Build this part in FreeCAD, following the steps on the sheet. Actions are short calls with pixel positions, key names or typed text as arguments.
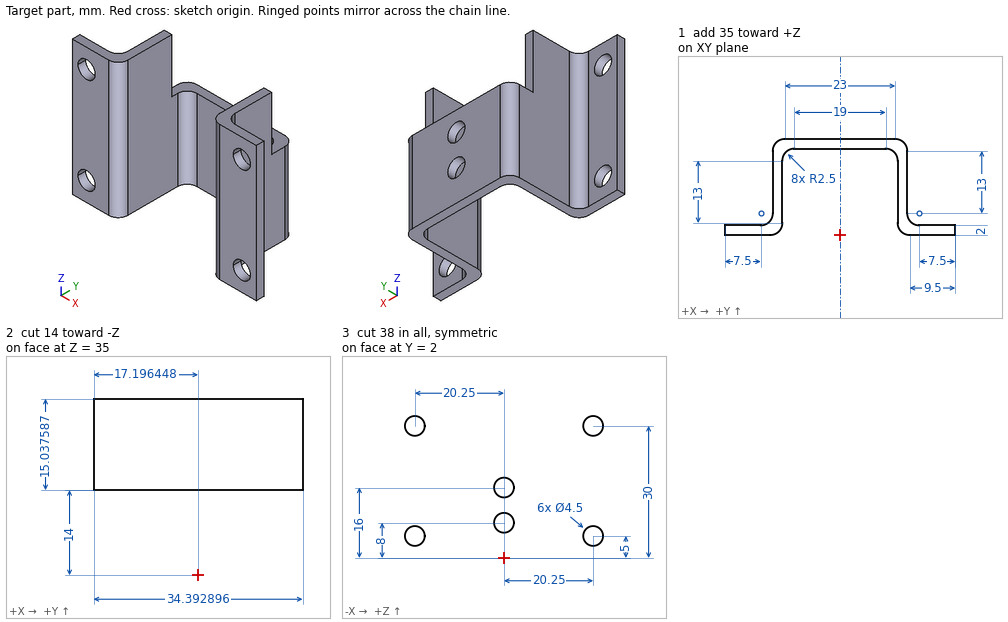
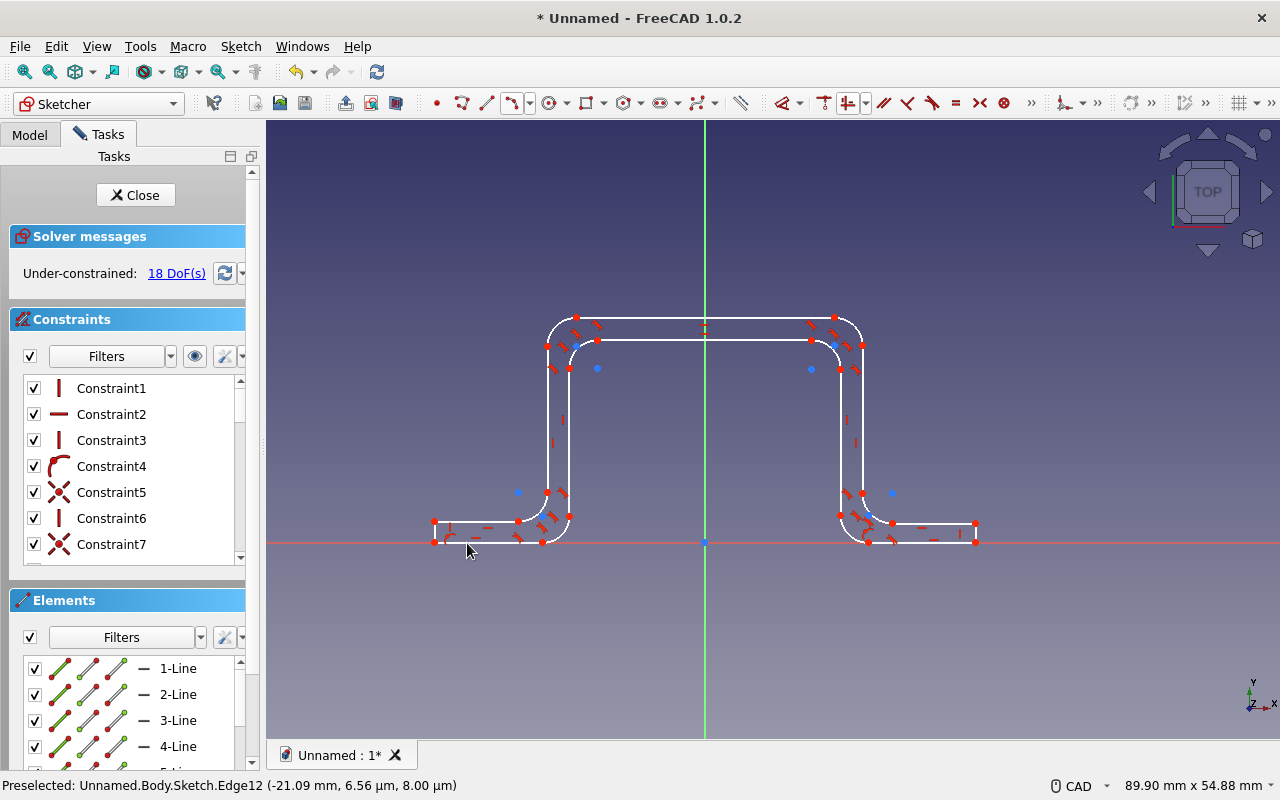
click(585, 343)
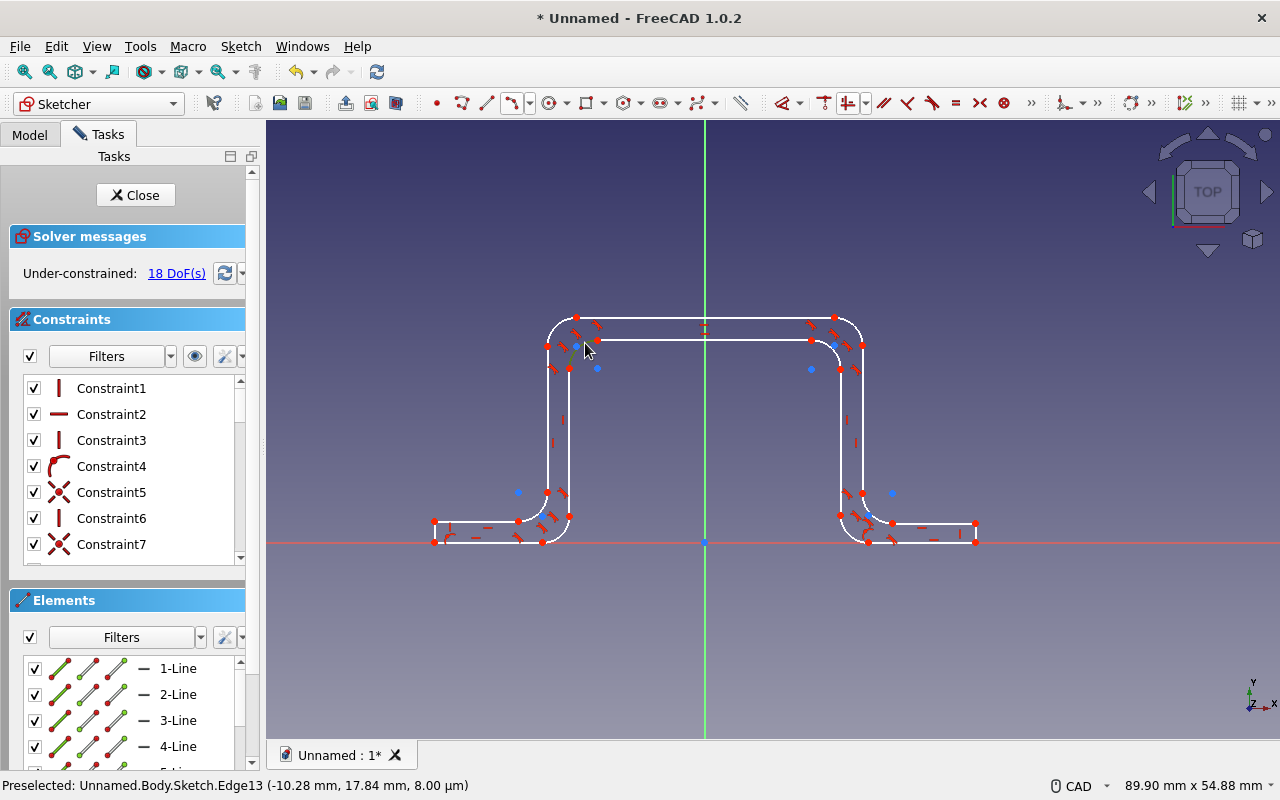
click(837, 356)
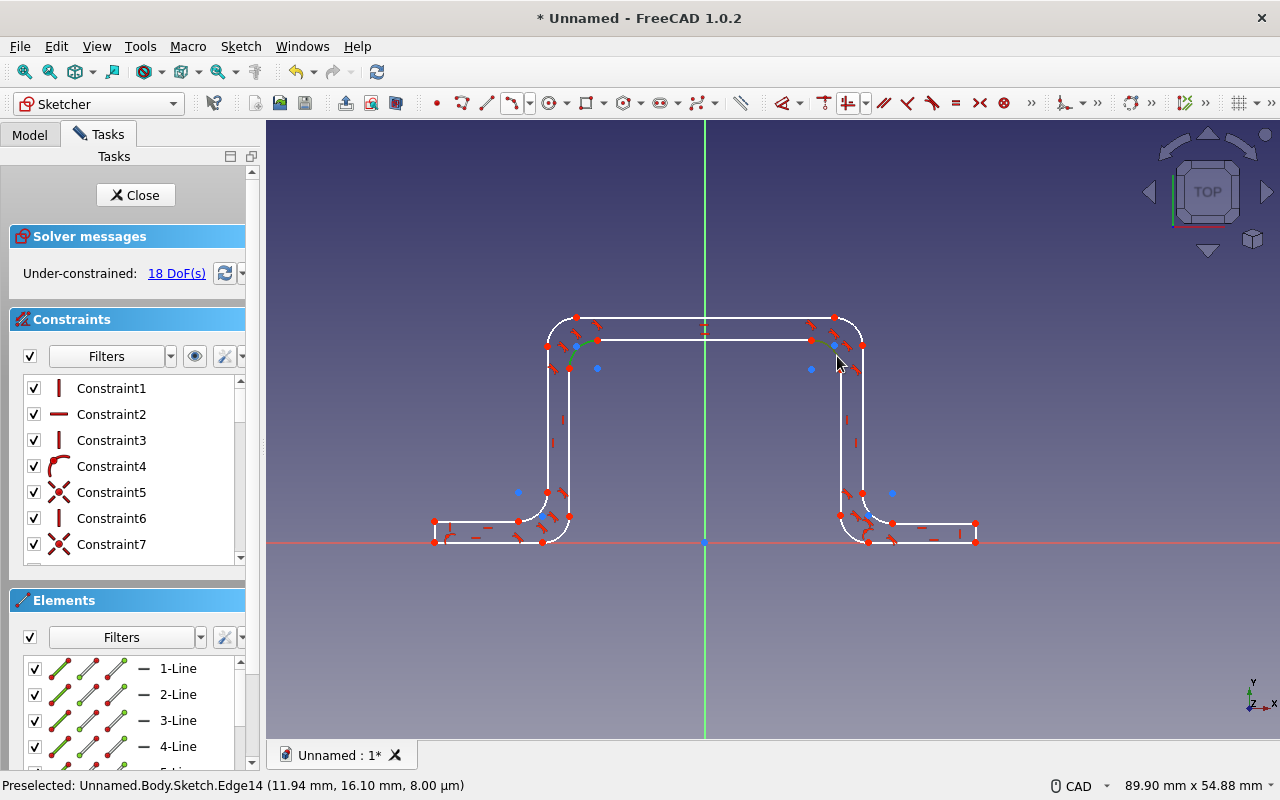
click(844, 528)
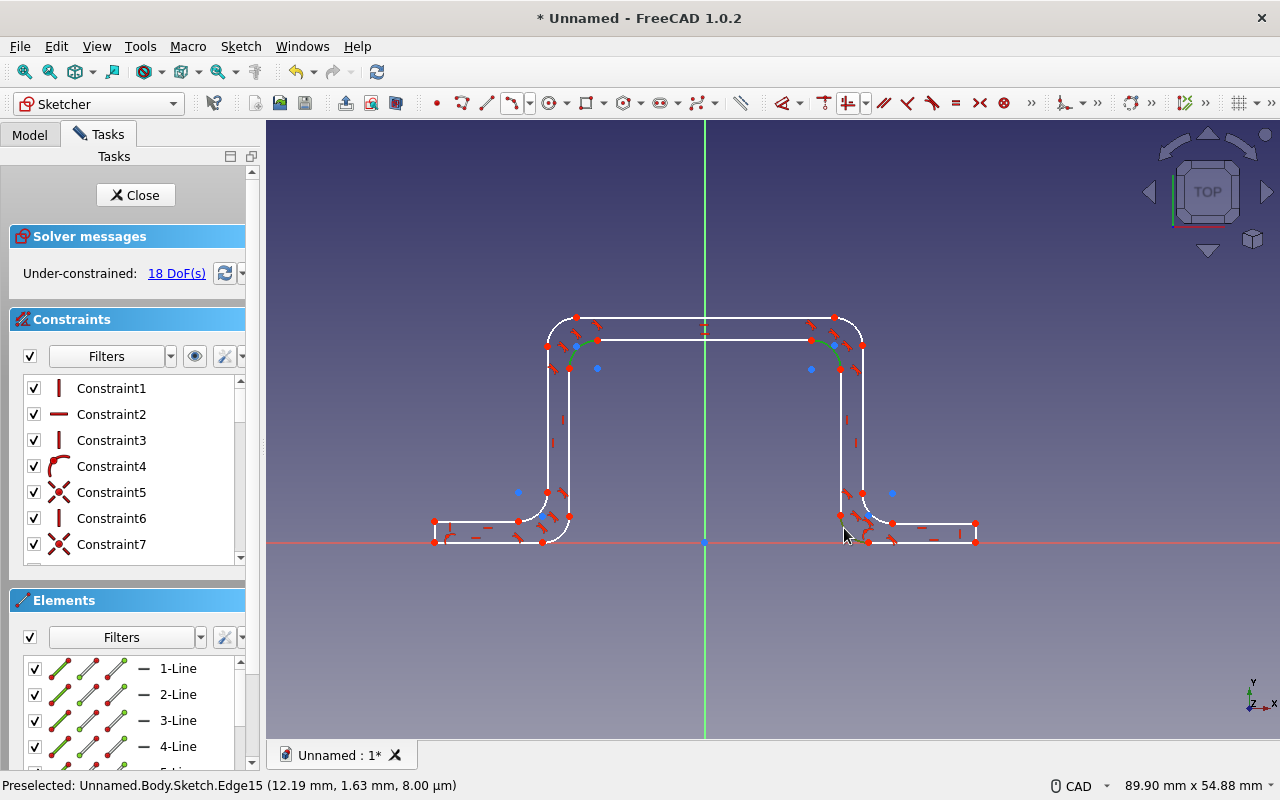
click(866, 507)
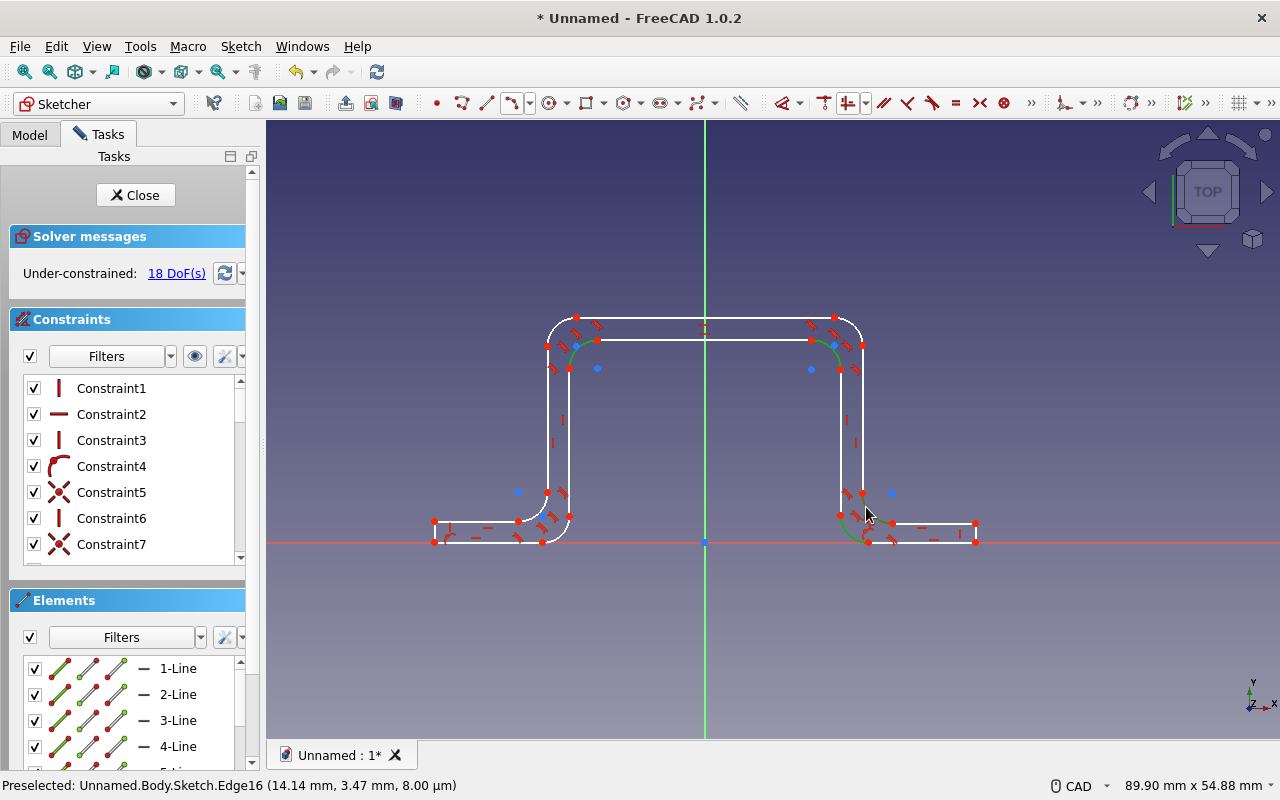
click(859, 333)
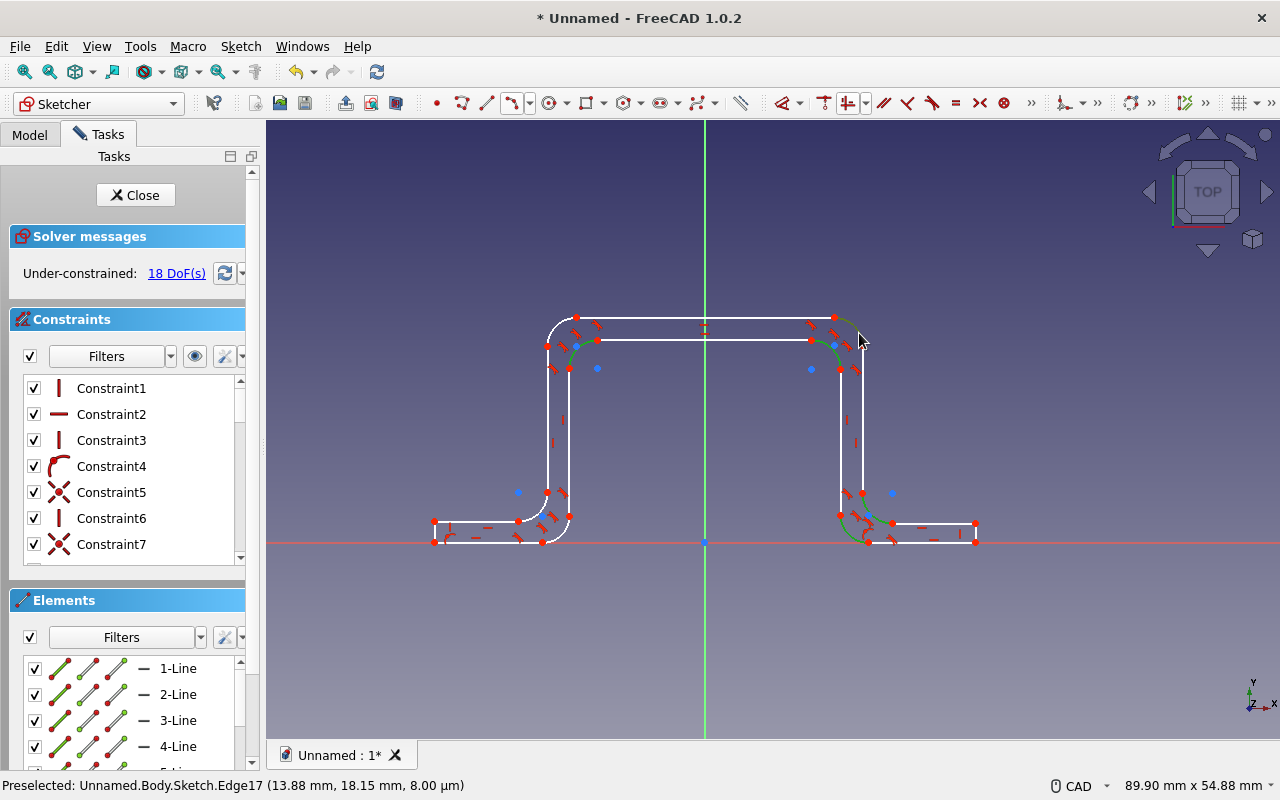
click(563, 321)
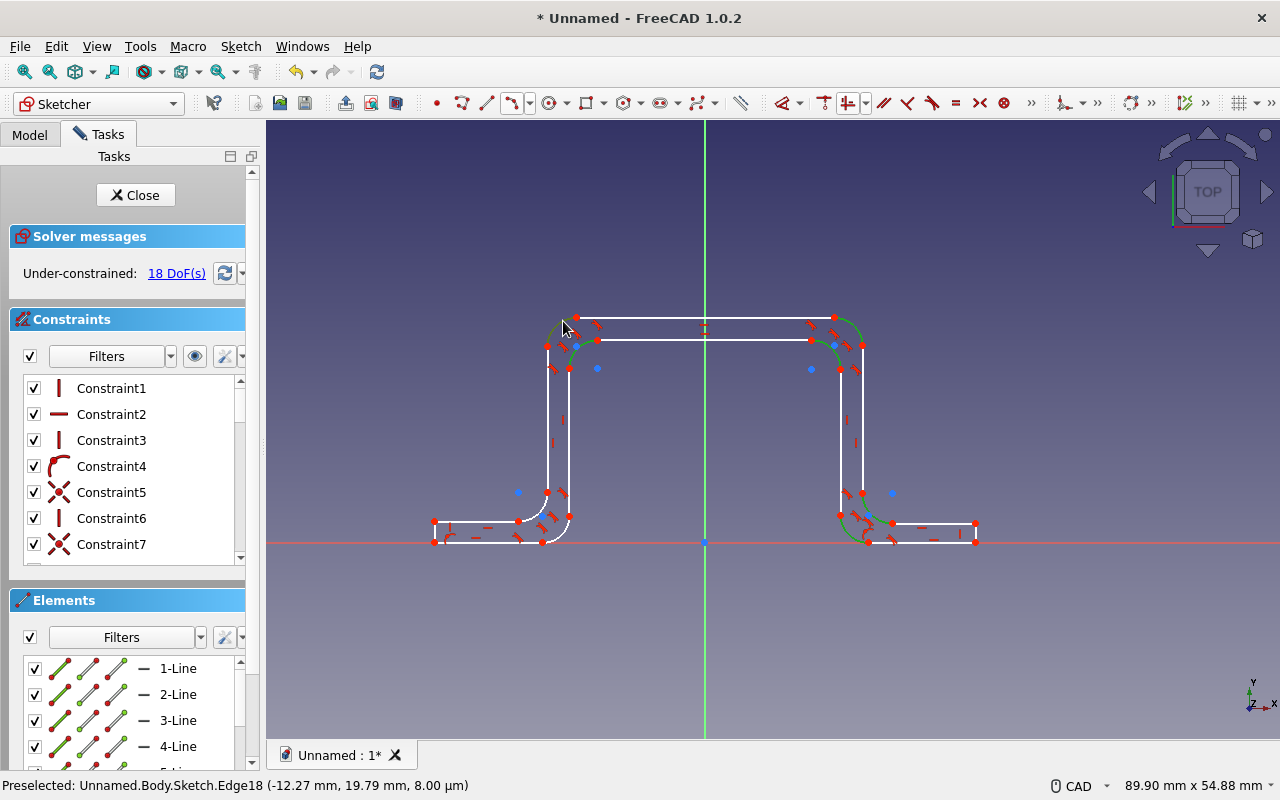
click(532, 518)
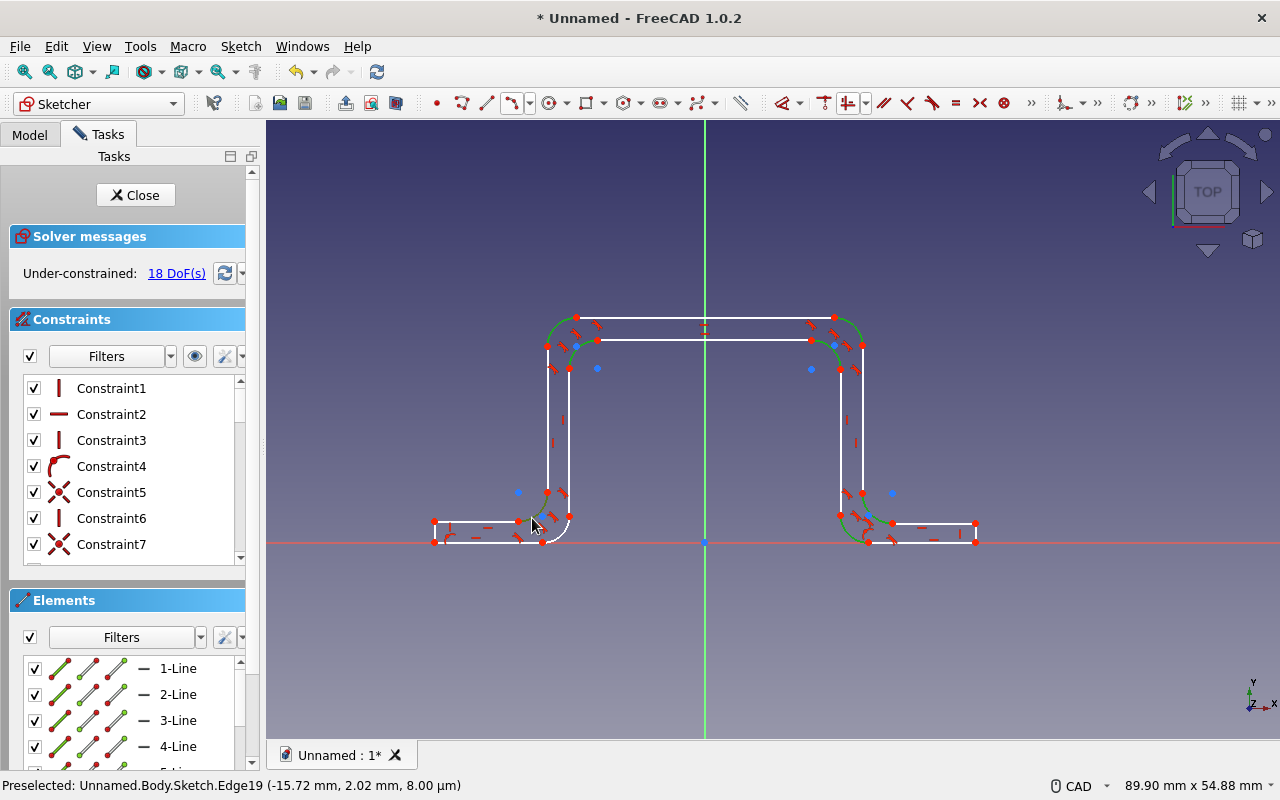
click(555, 540)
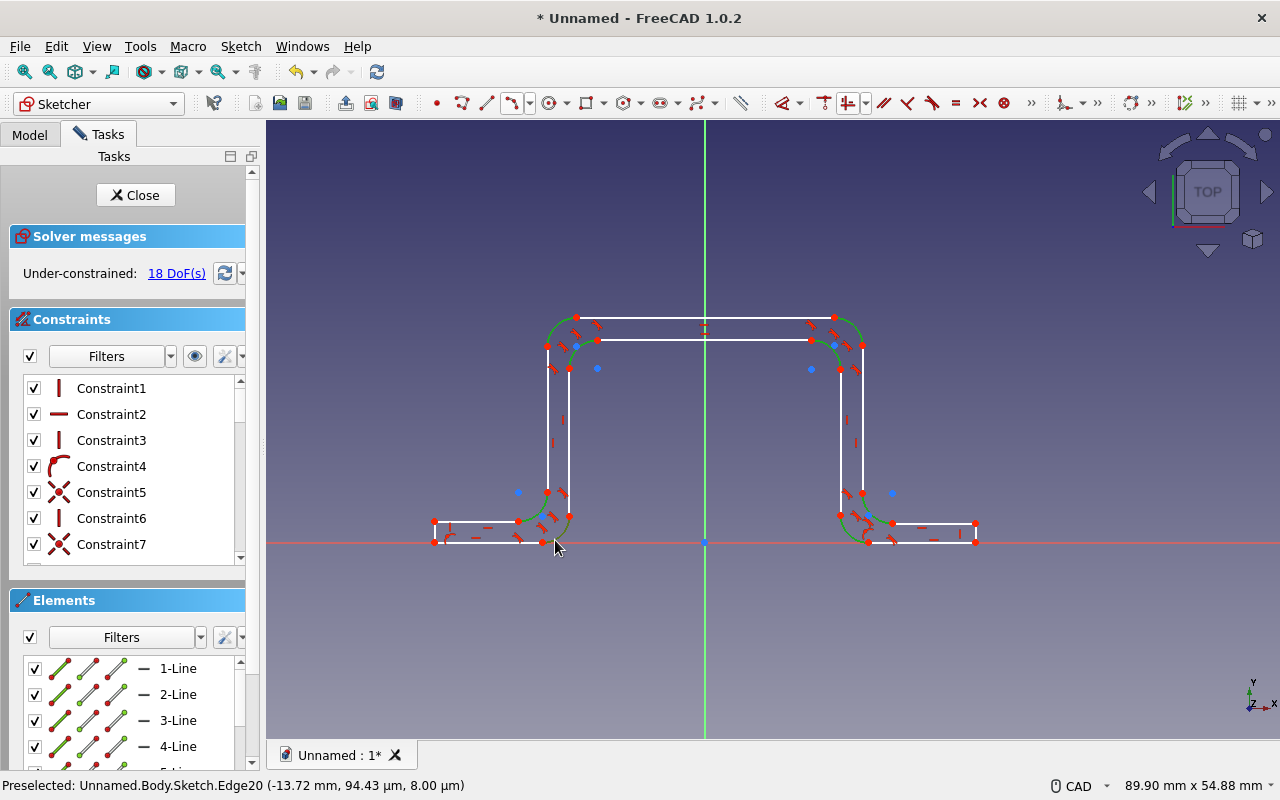
click(956, 104)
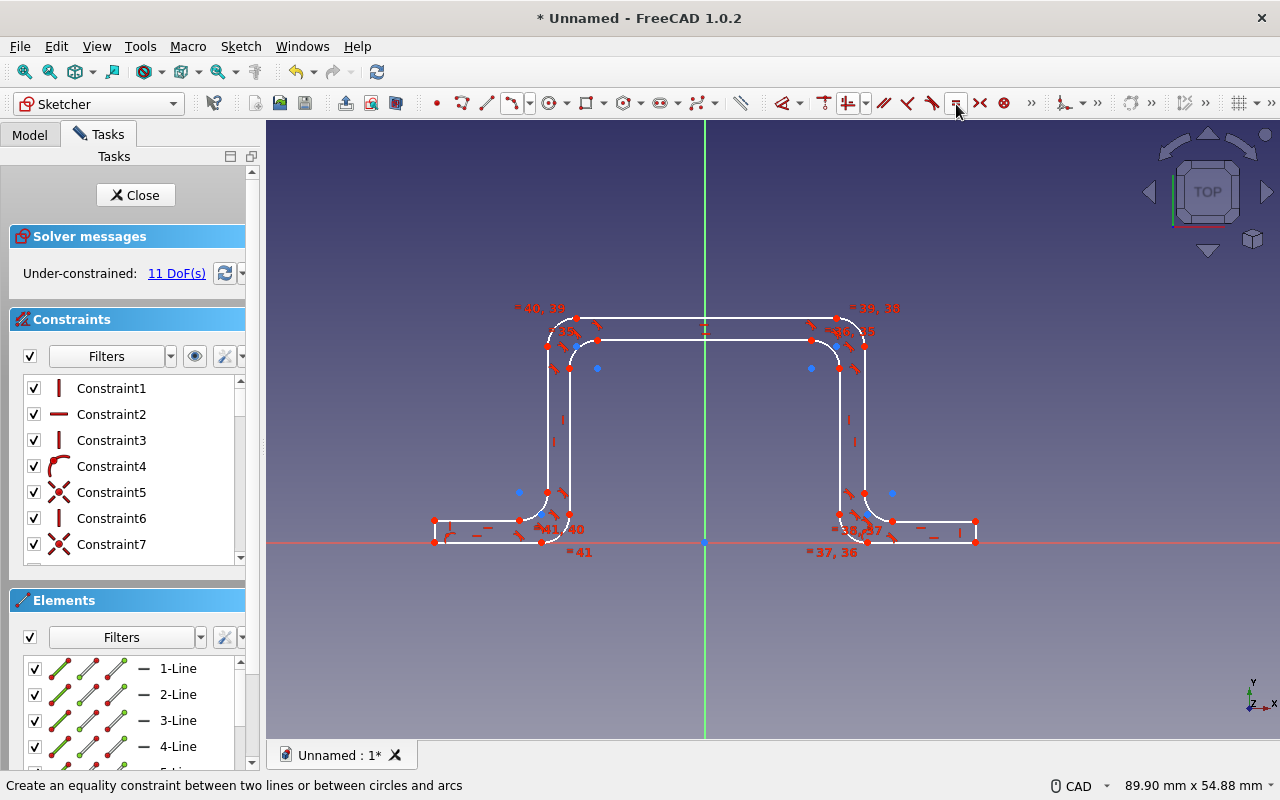
click(893, 494)